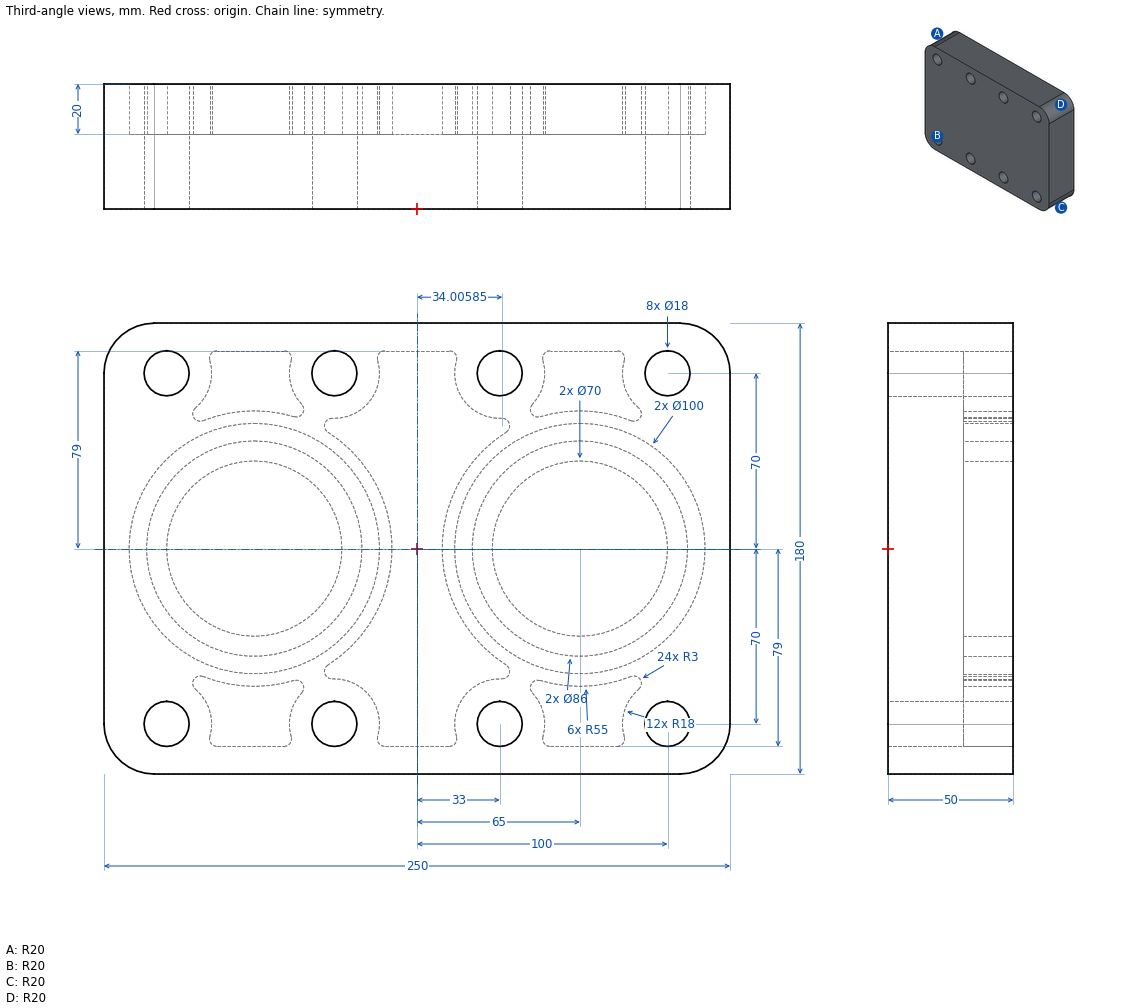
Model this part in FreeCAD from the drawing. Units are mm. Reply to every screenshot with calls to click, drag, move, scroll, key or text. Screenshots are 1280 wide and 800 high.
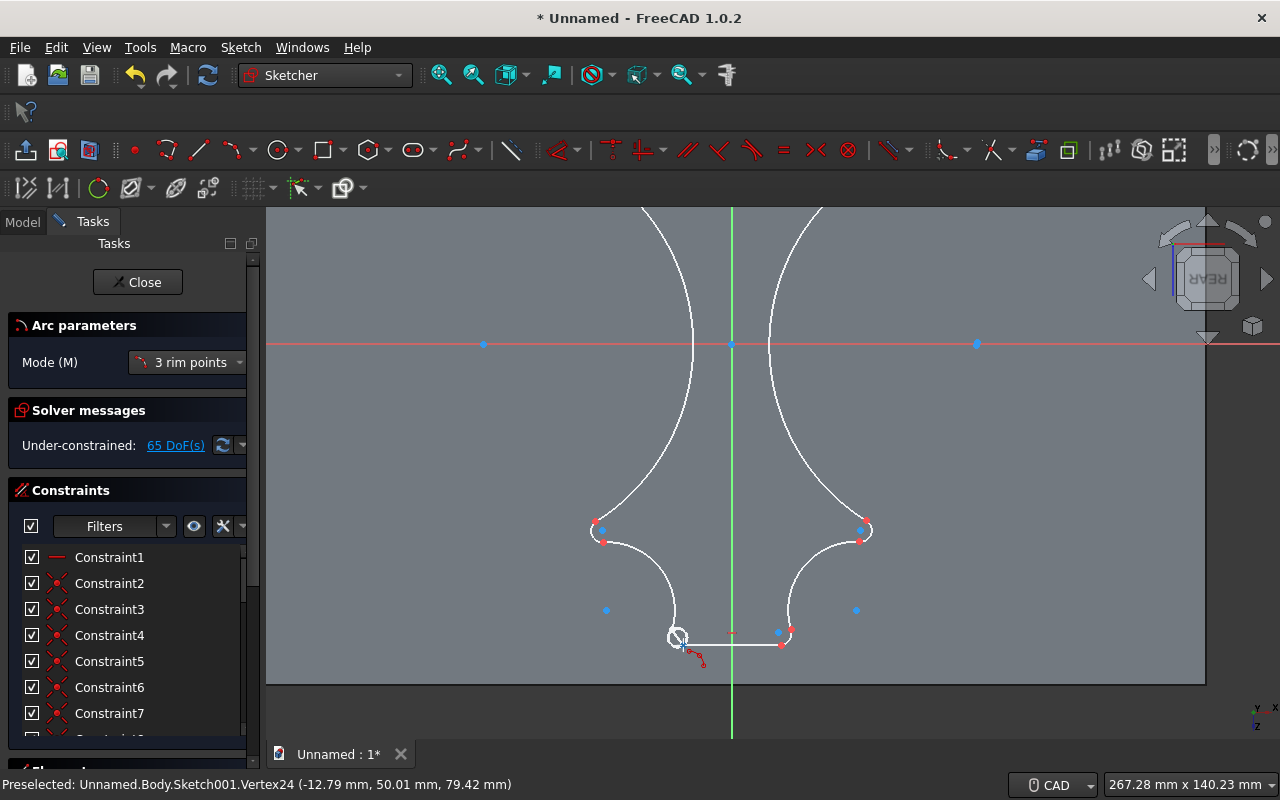
scroll(674, 639, up, 7)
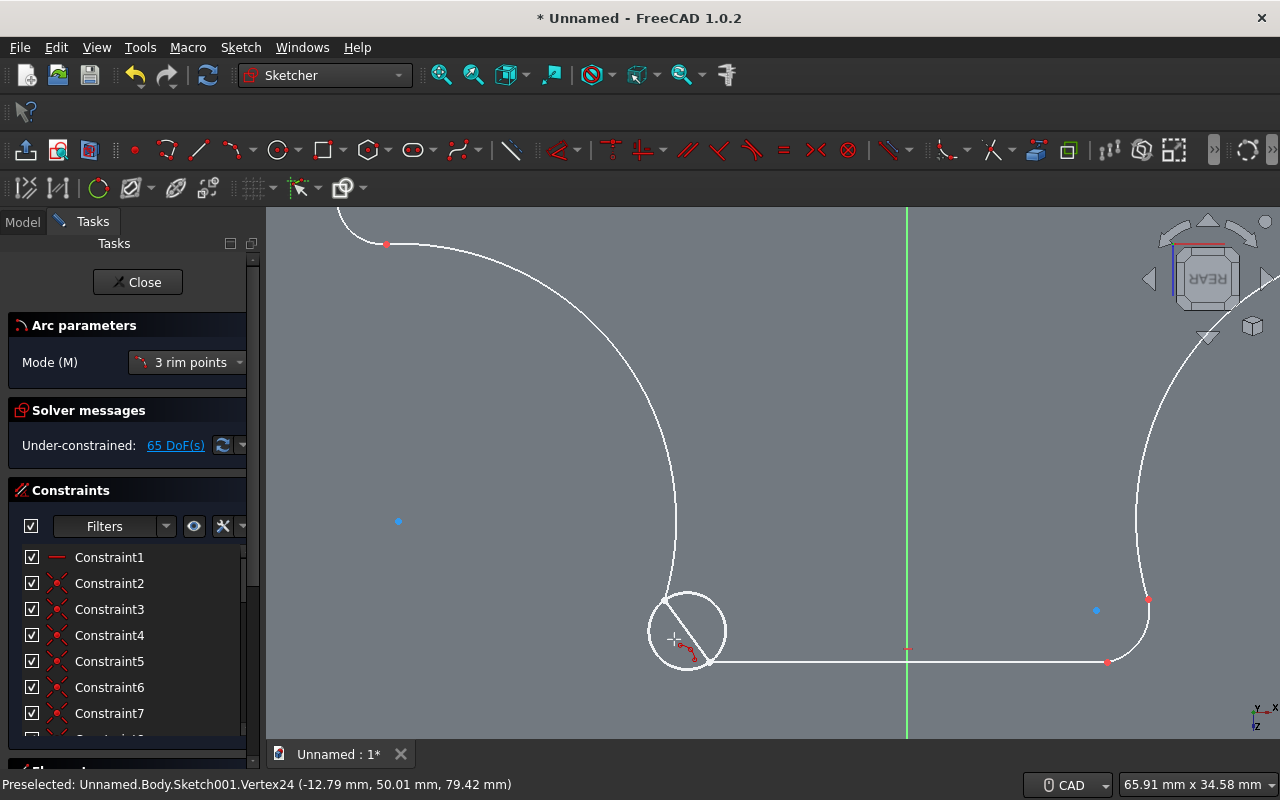
click(671, 637)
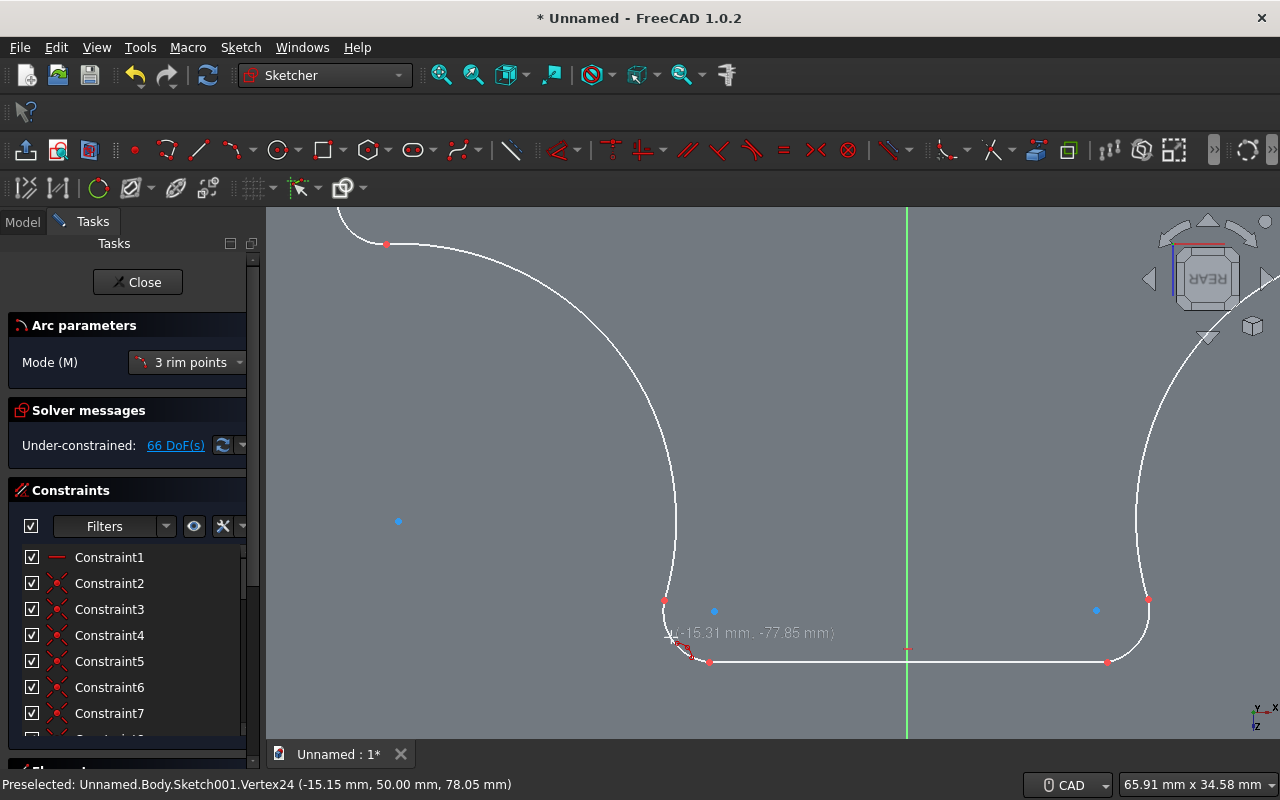
click(200, 150)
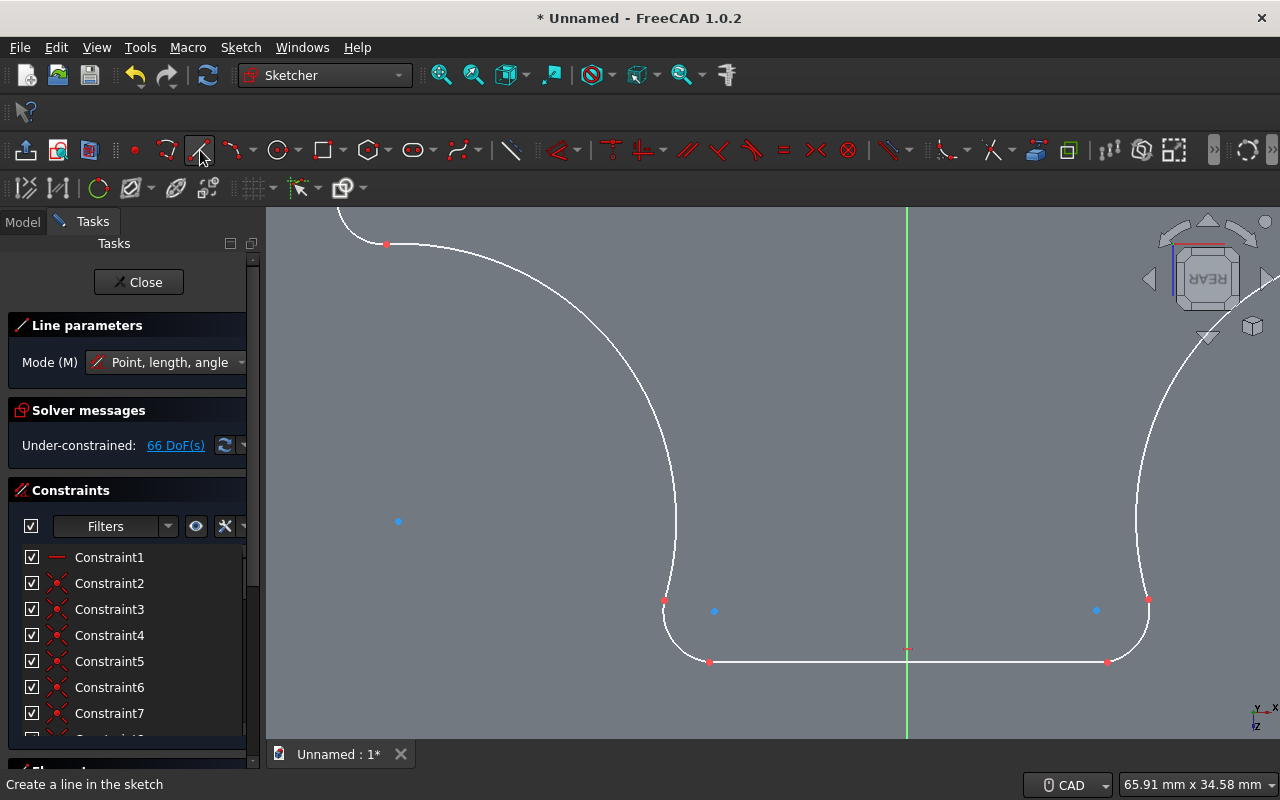
scroll(673, 635, down, 10)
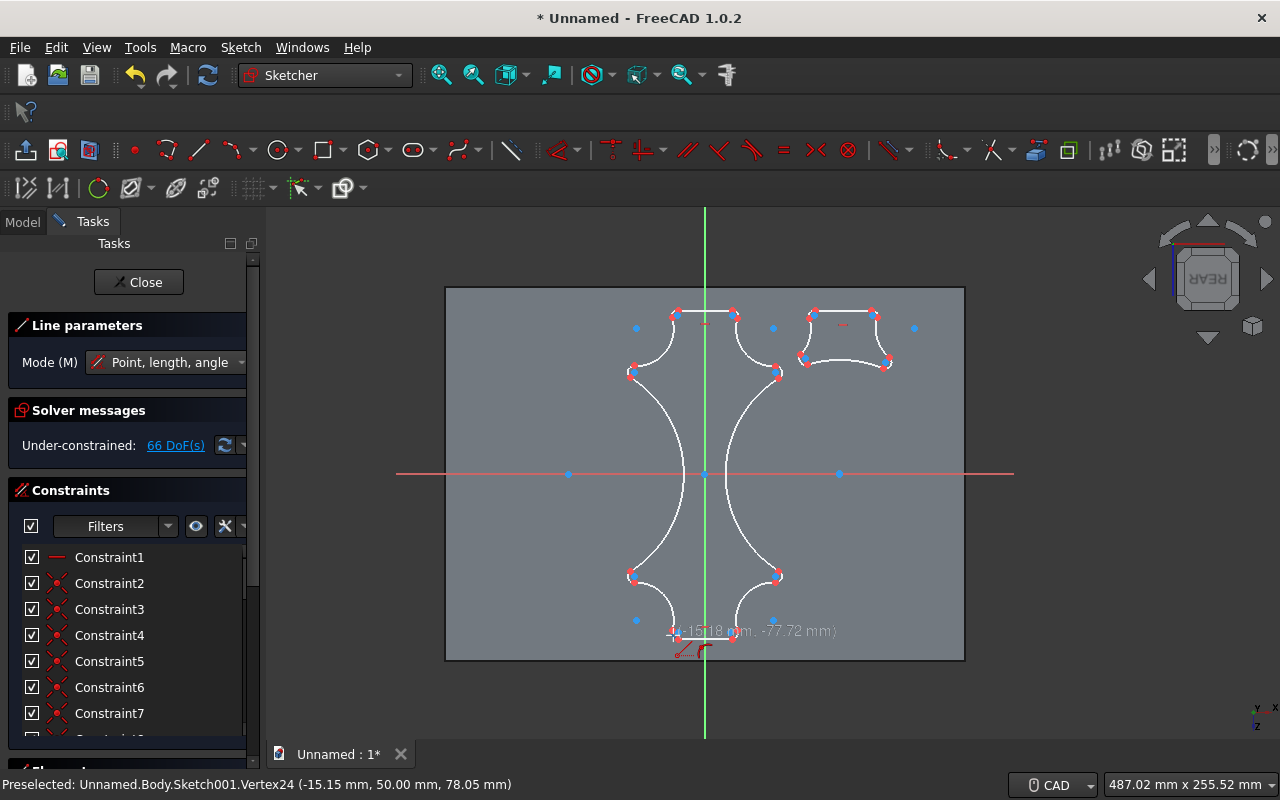
click(594, 310)
click(539, 310)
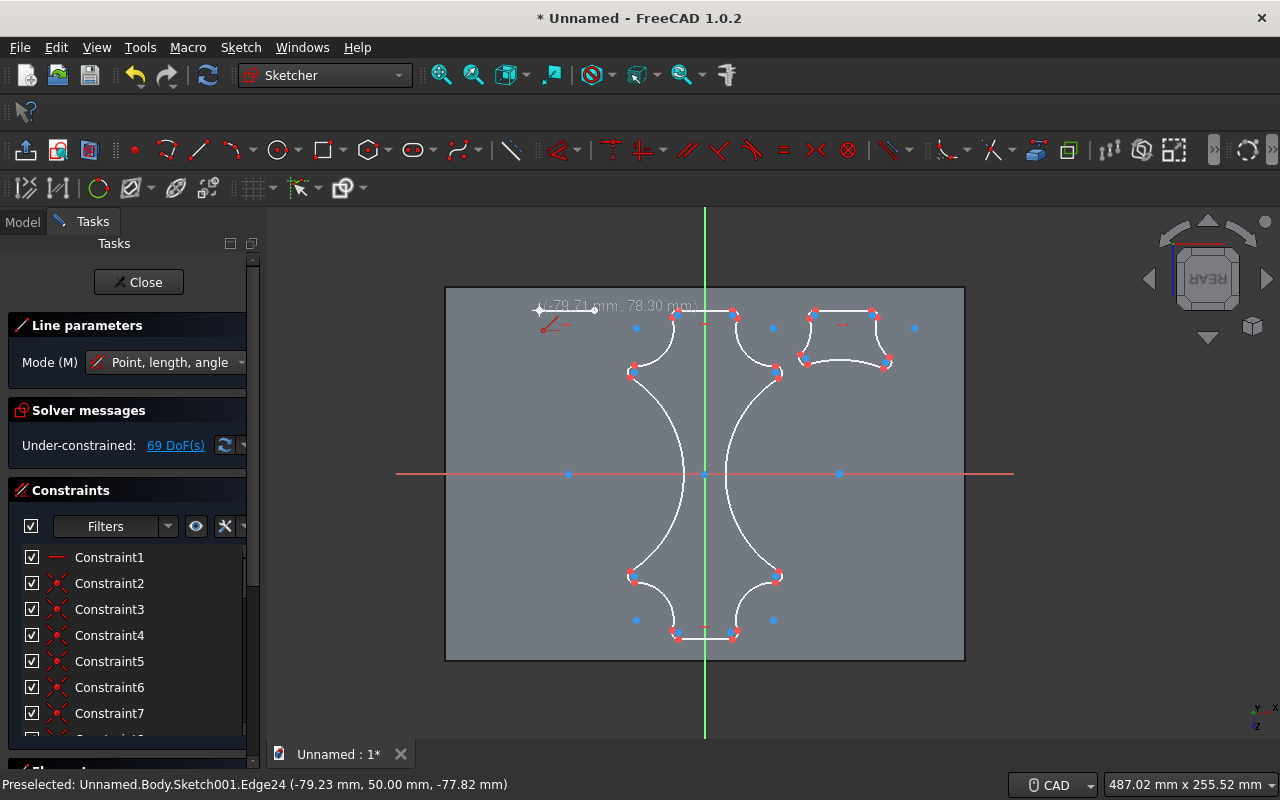
click(232, 150)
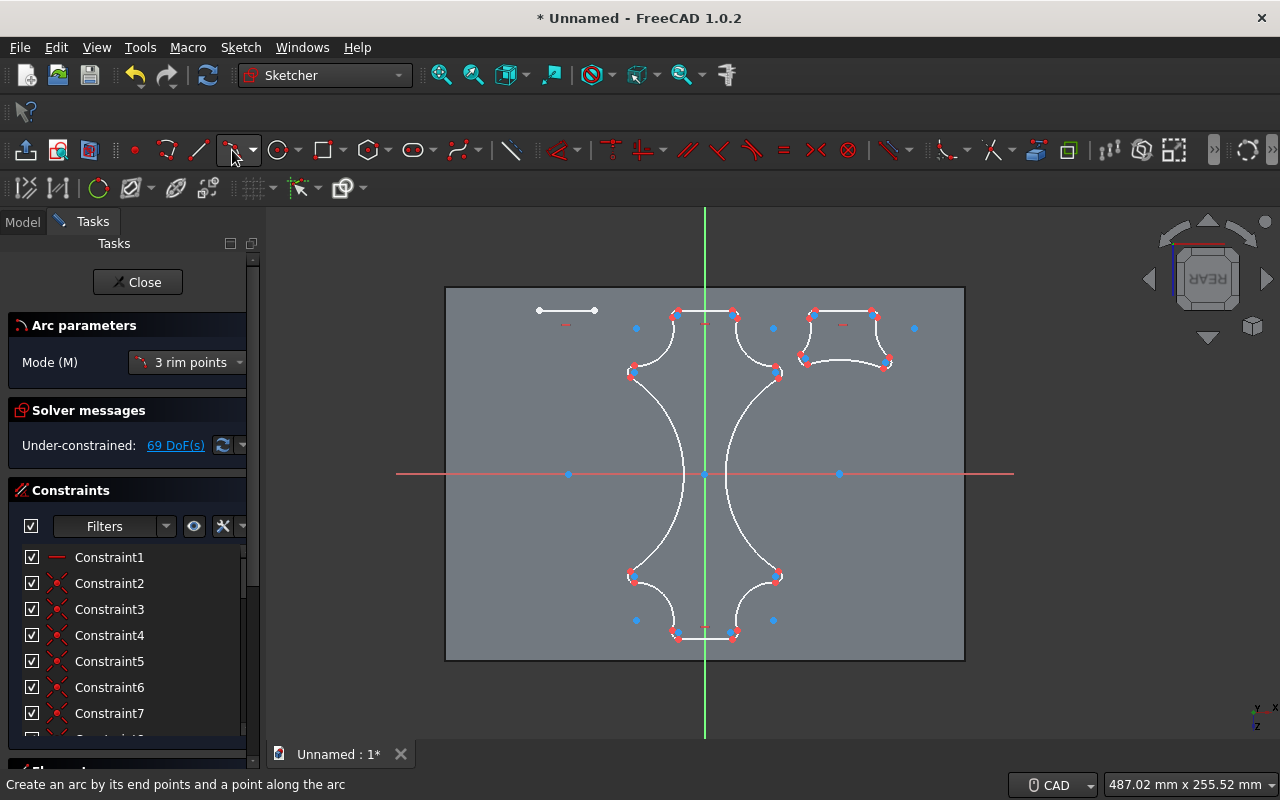
click(539, 311)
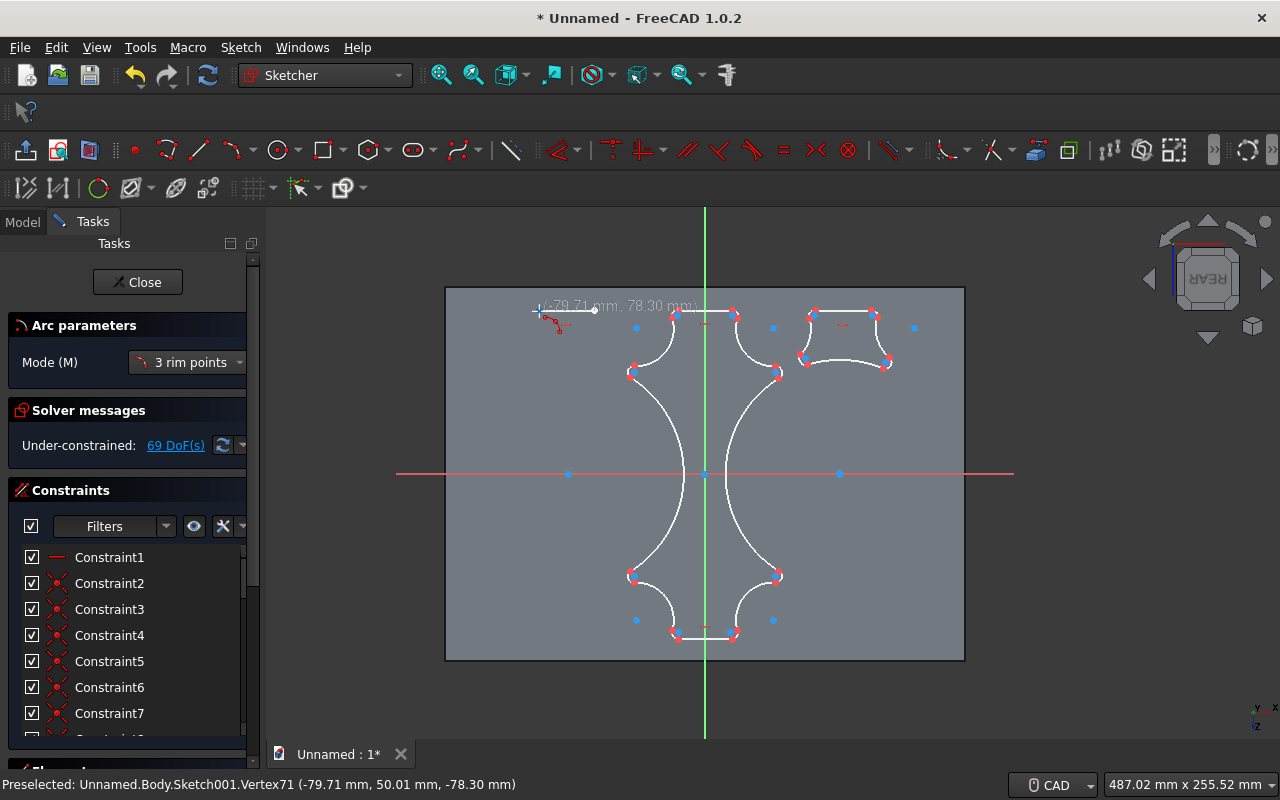
scroll(533, 318, up, 3)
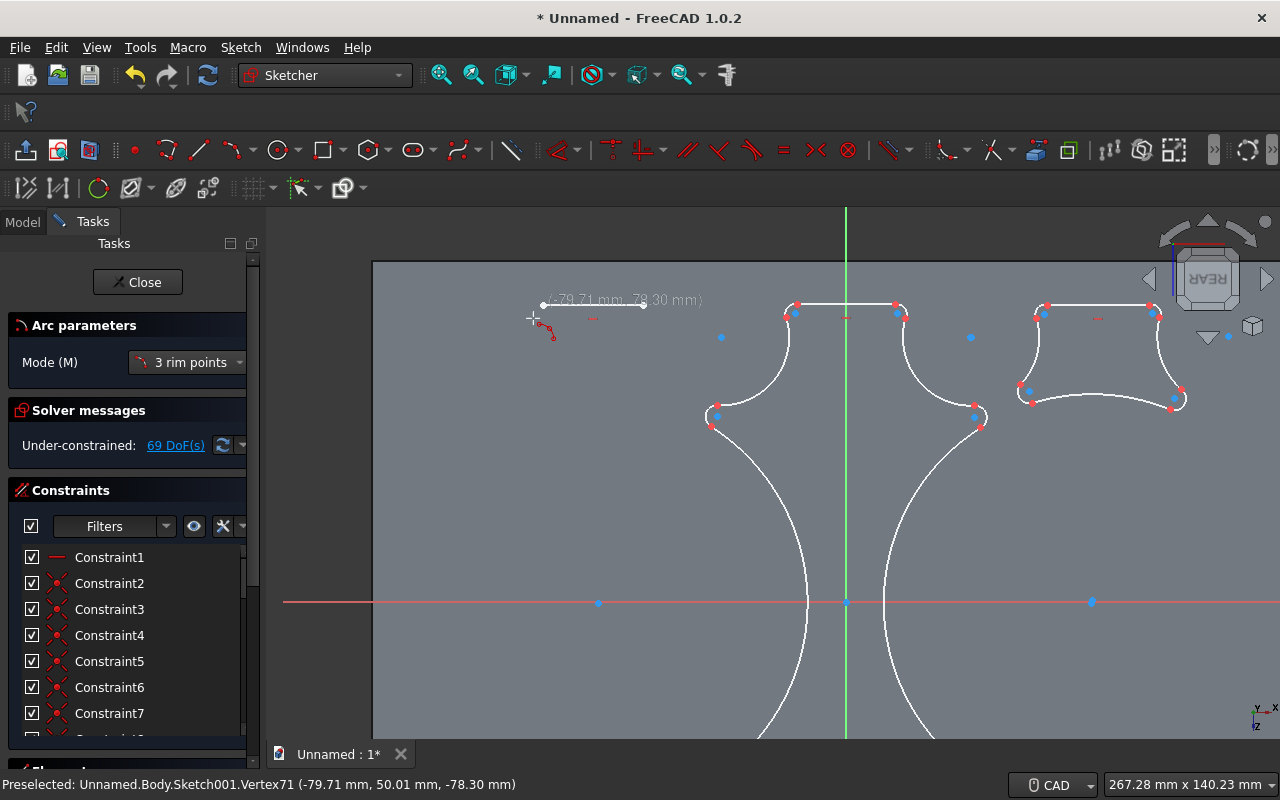
click(532, 317)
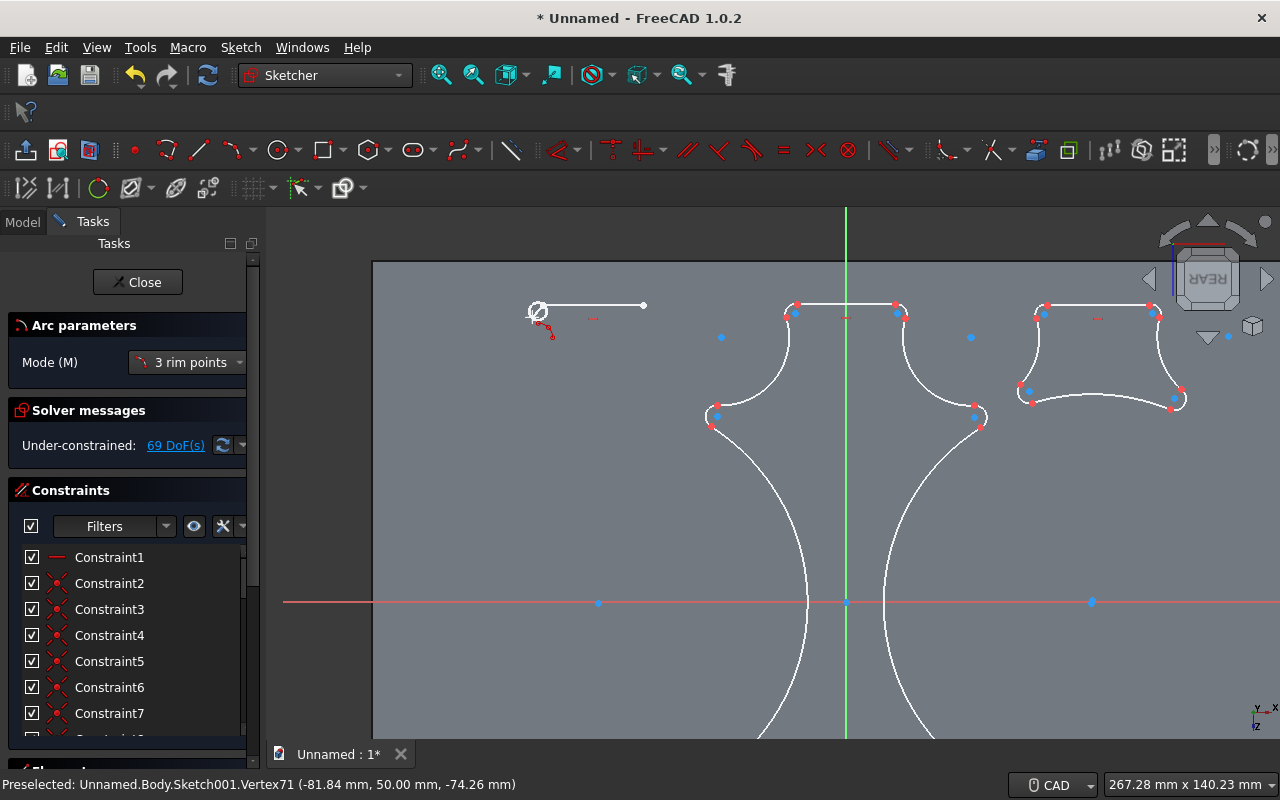
scroll(534, 307, up, 7)